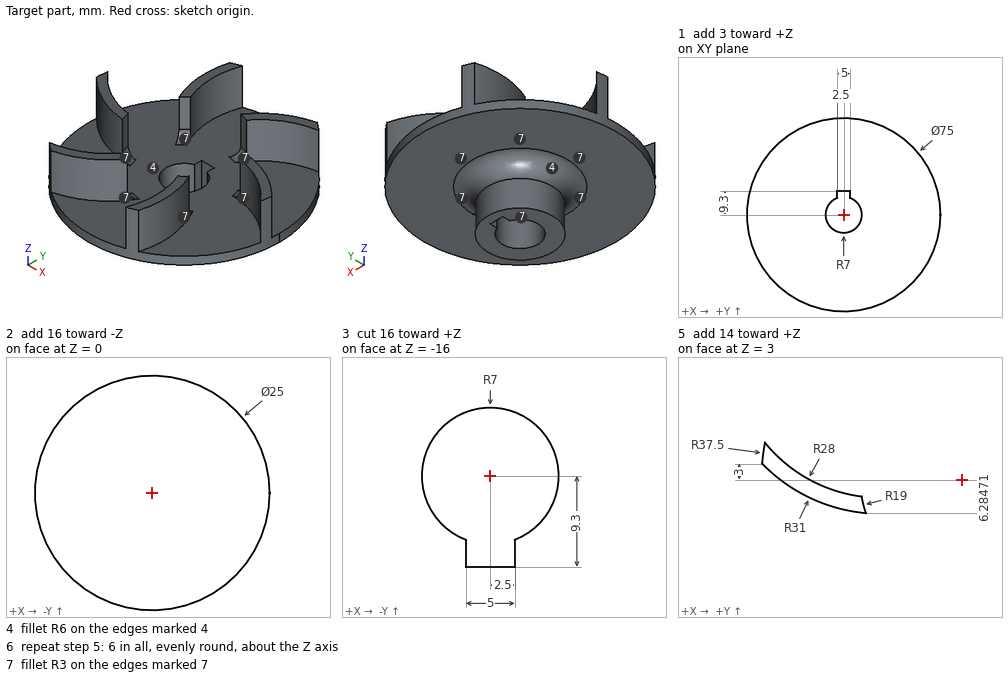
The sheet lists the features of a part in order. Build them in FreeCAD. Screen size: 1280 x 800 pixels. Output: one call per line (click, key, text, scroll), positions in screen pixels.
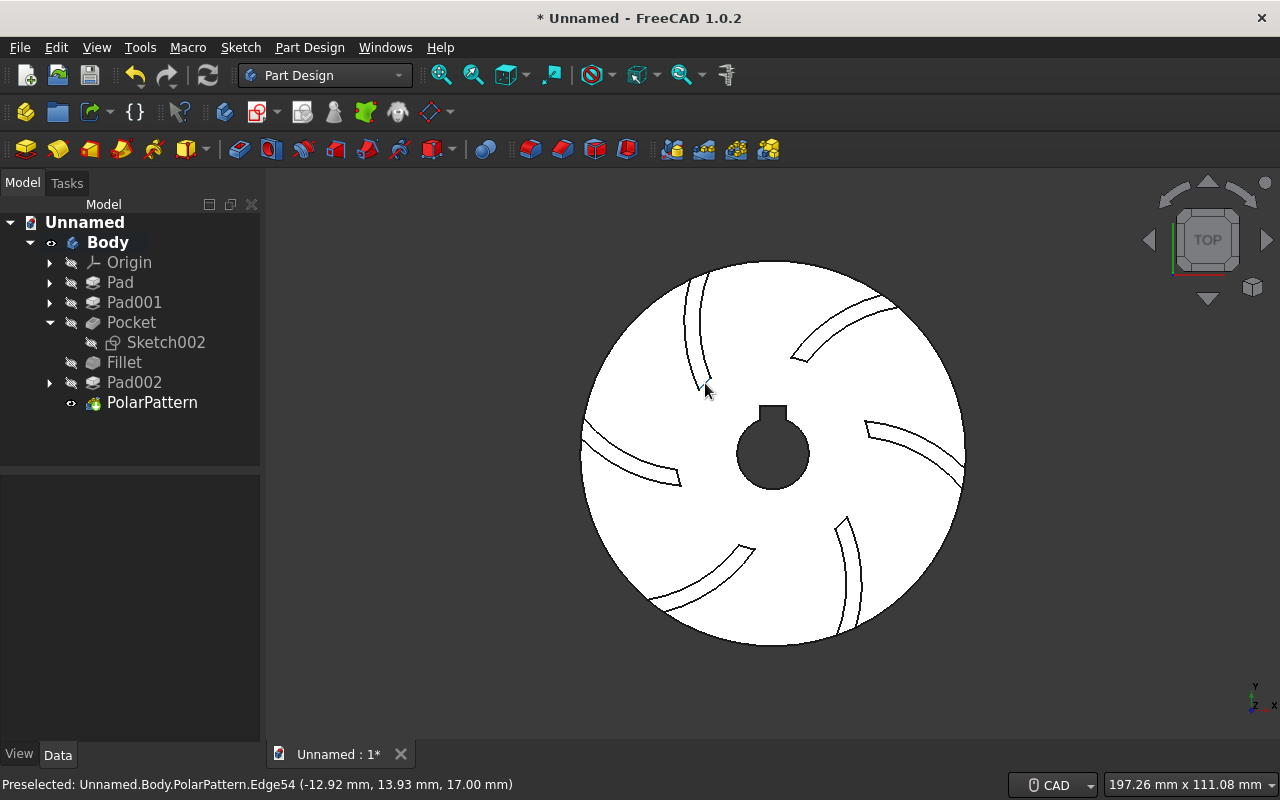
key(0)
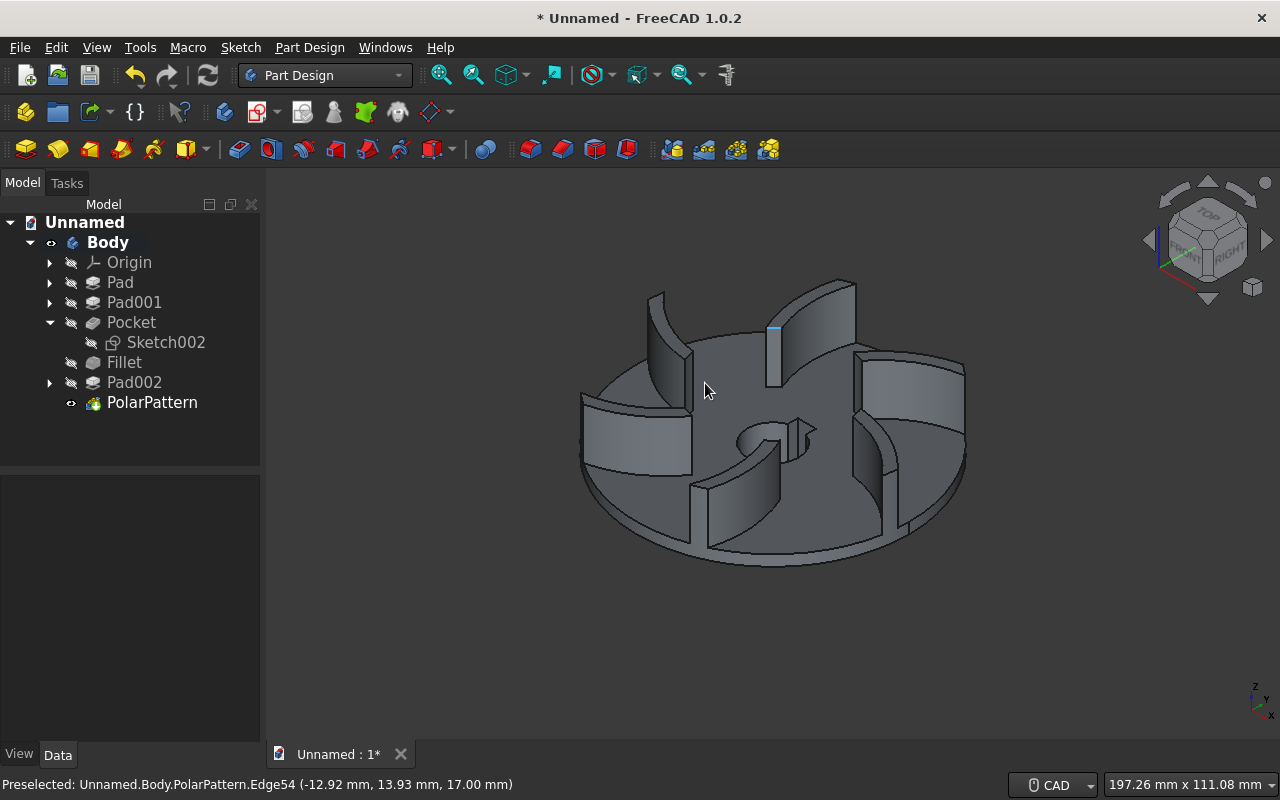
scroll(774, 386, up, 5)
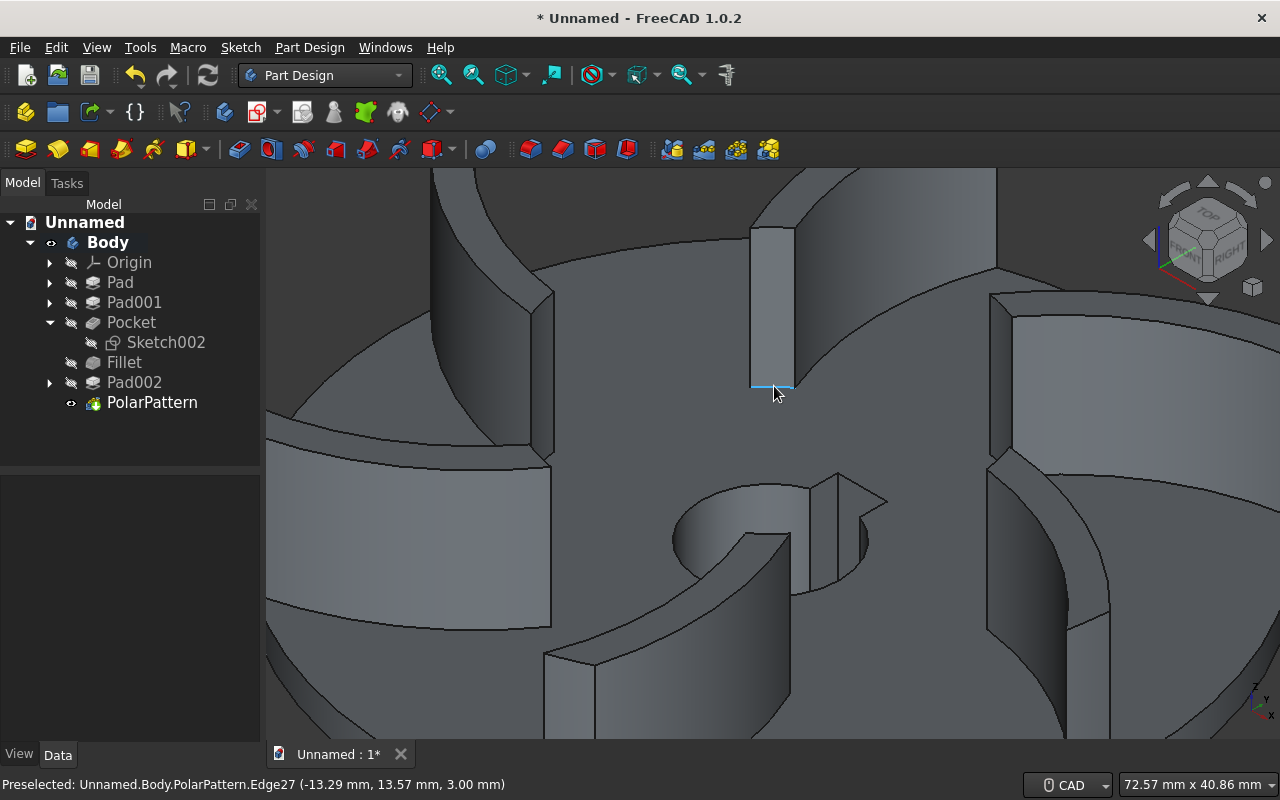
key(v)
key(f)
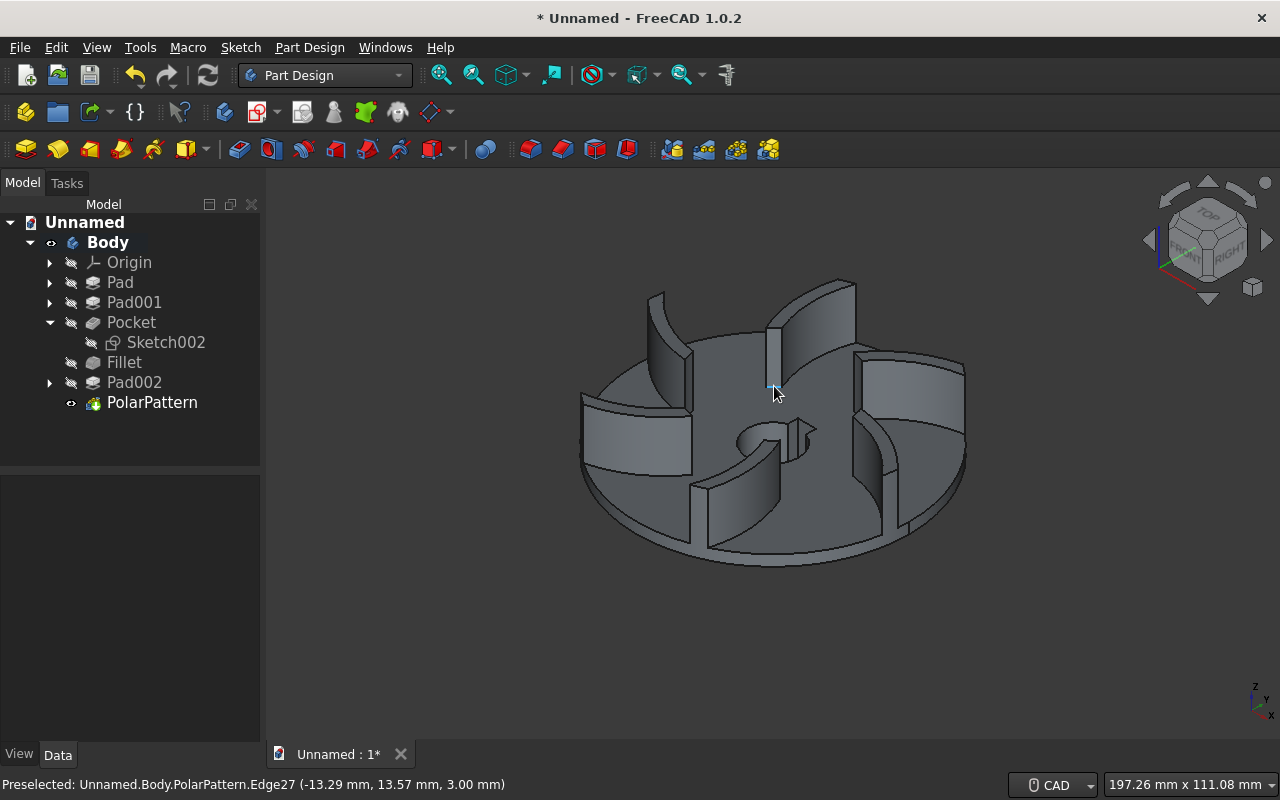
key(1)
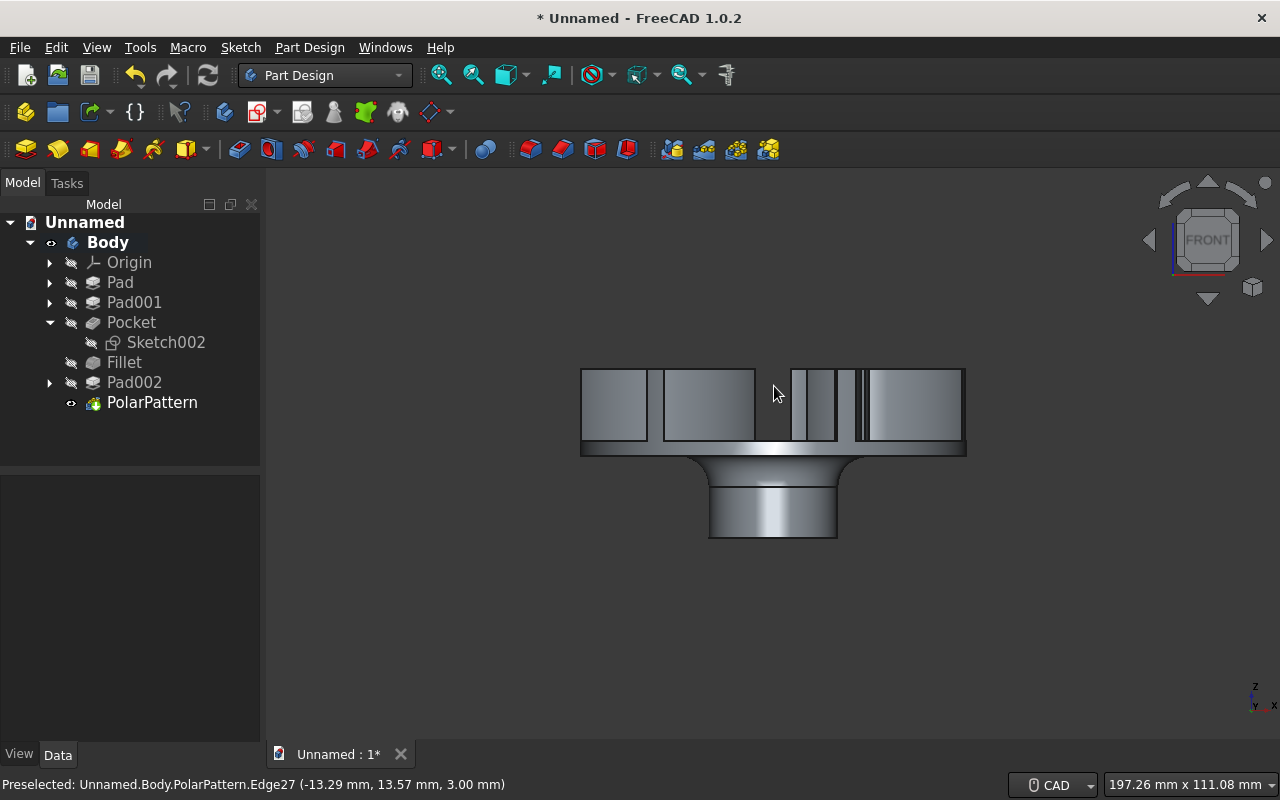
key(v)
key(f)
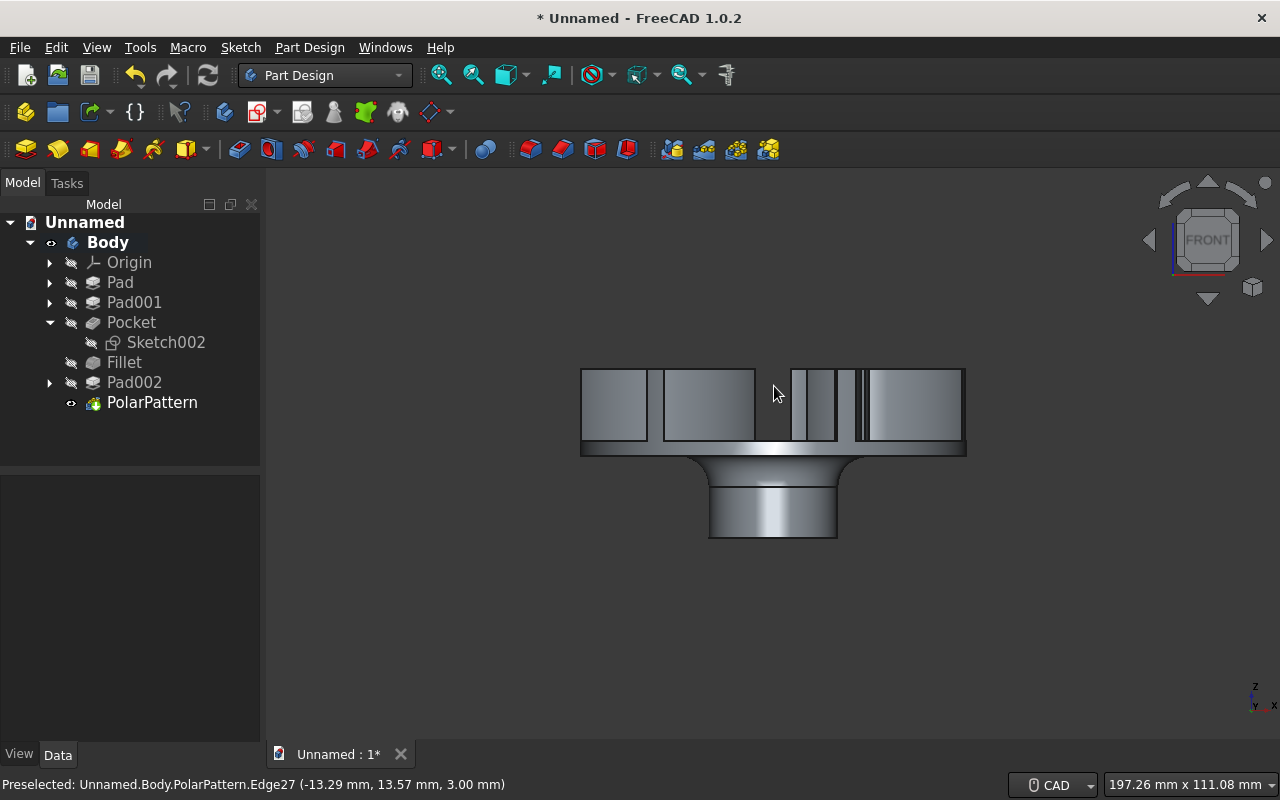
scroll(705, 440, up, 5)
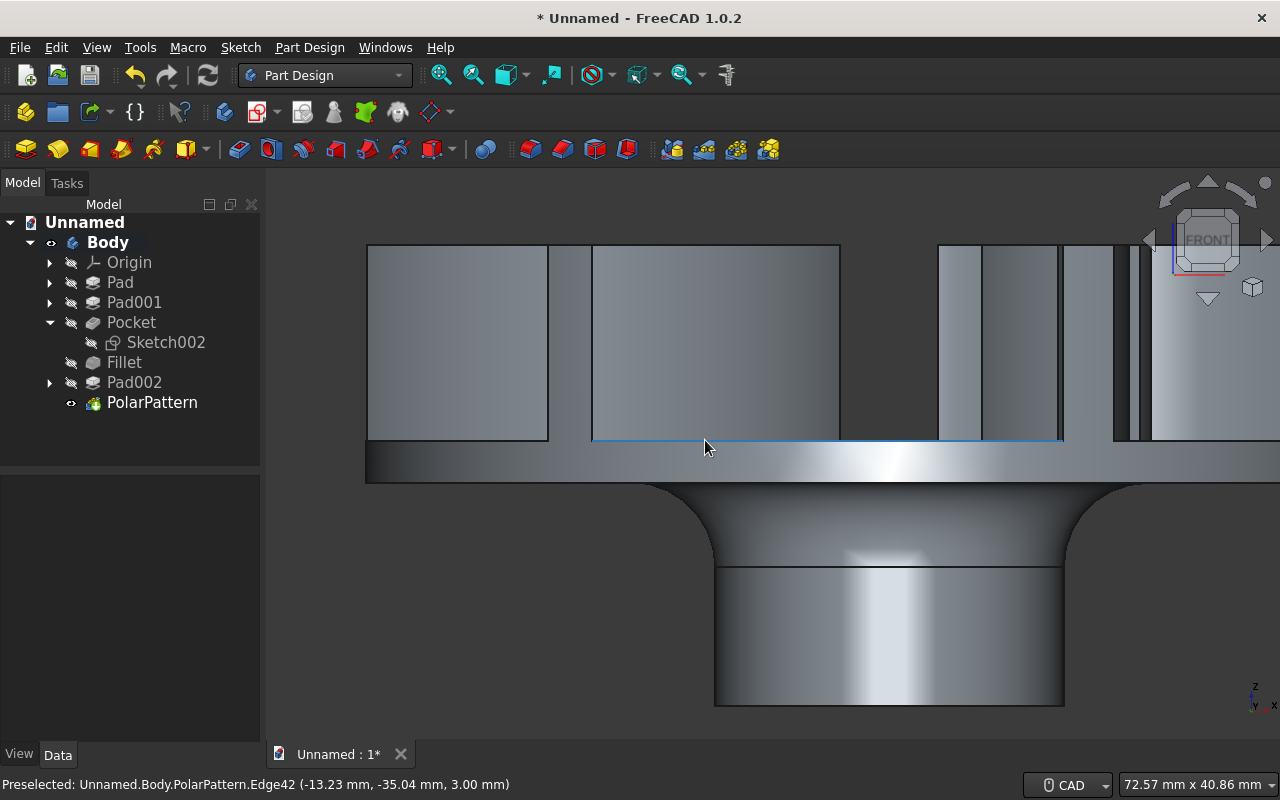
click(442, 76)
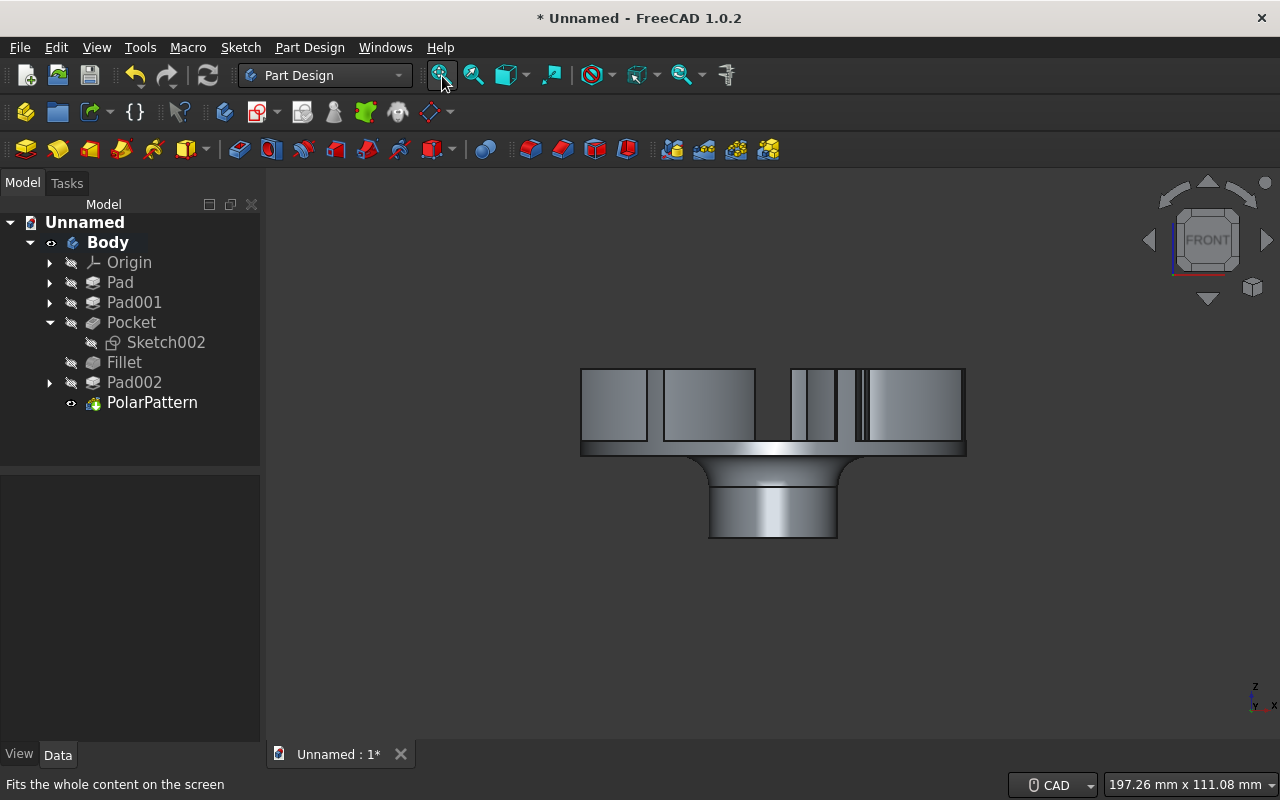
key(3)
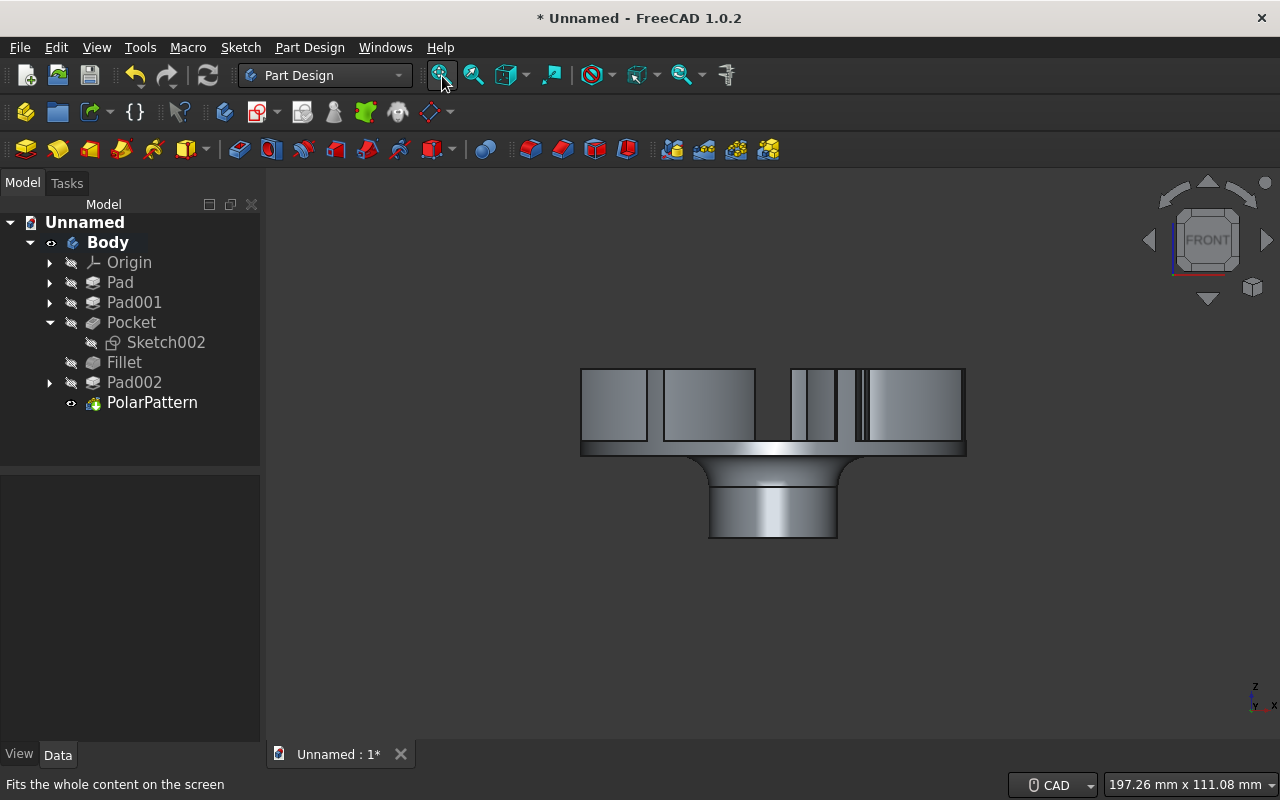
key(v)
key(f)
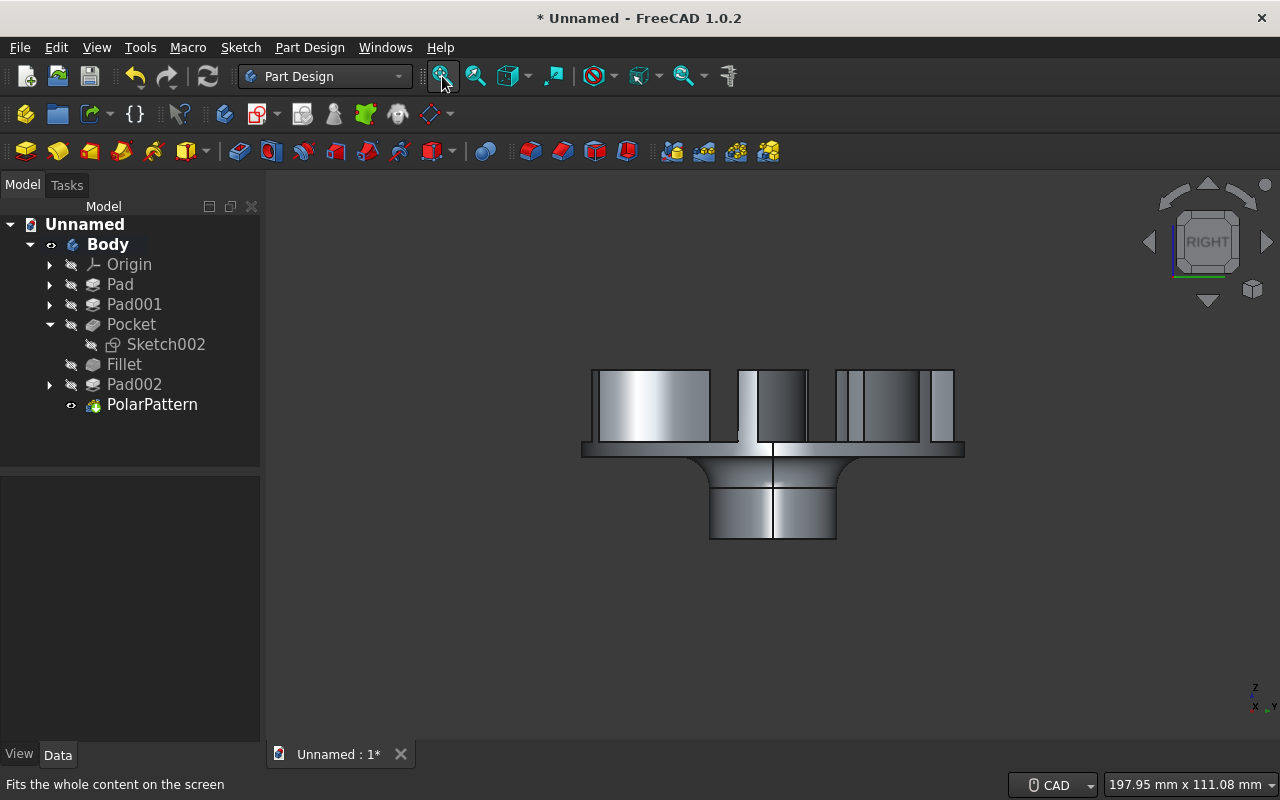
scroll(842, 441, up, 5)